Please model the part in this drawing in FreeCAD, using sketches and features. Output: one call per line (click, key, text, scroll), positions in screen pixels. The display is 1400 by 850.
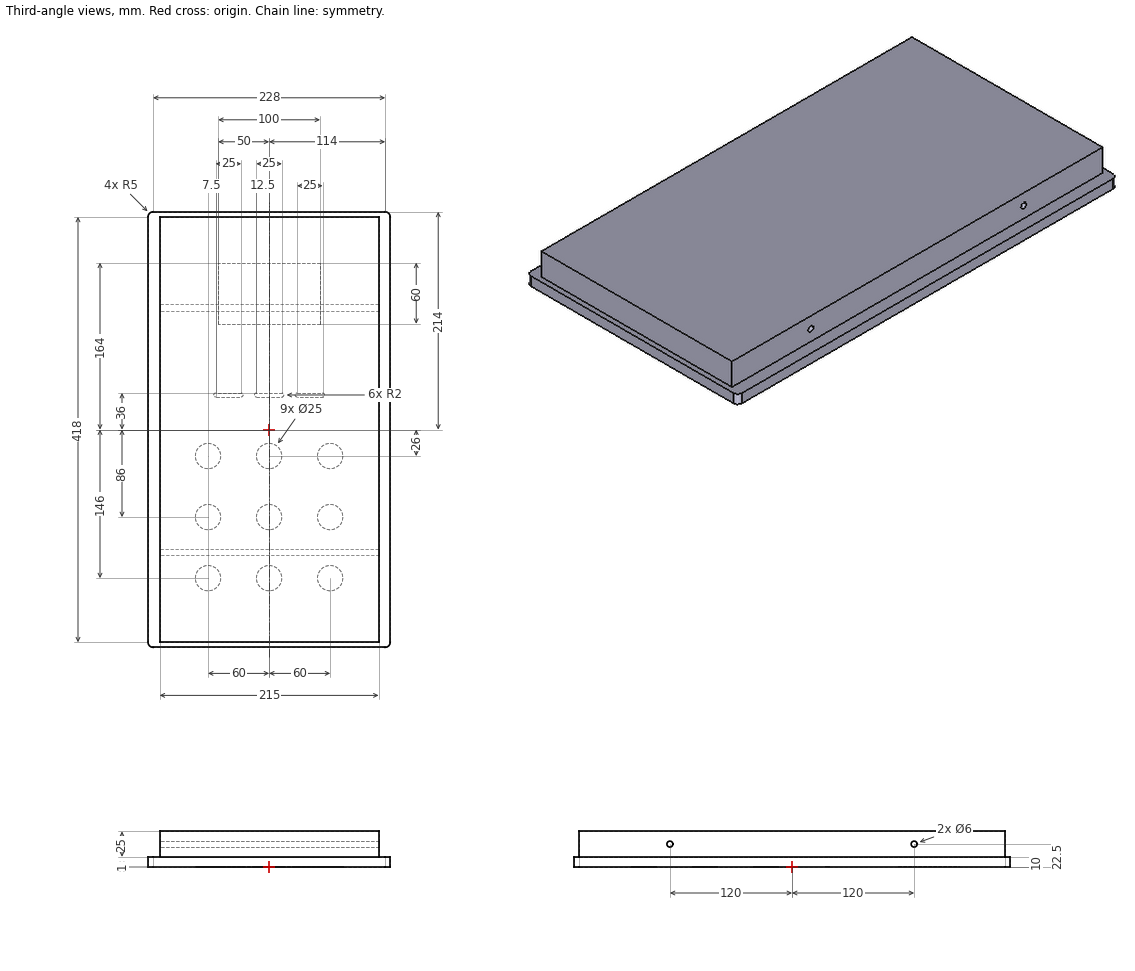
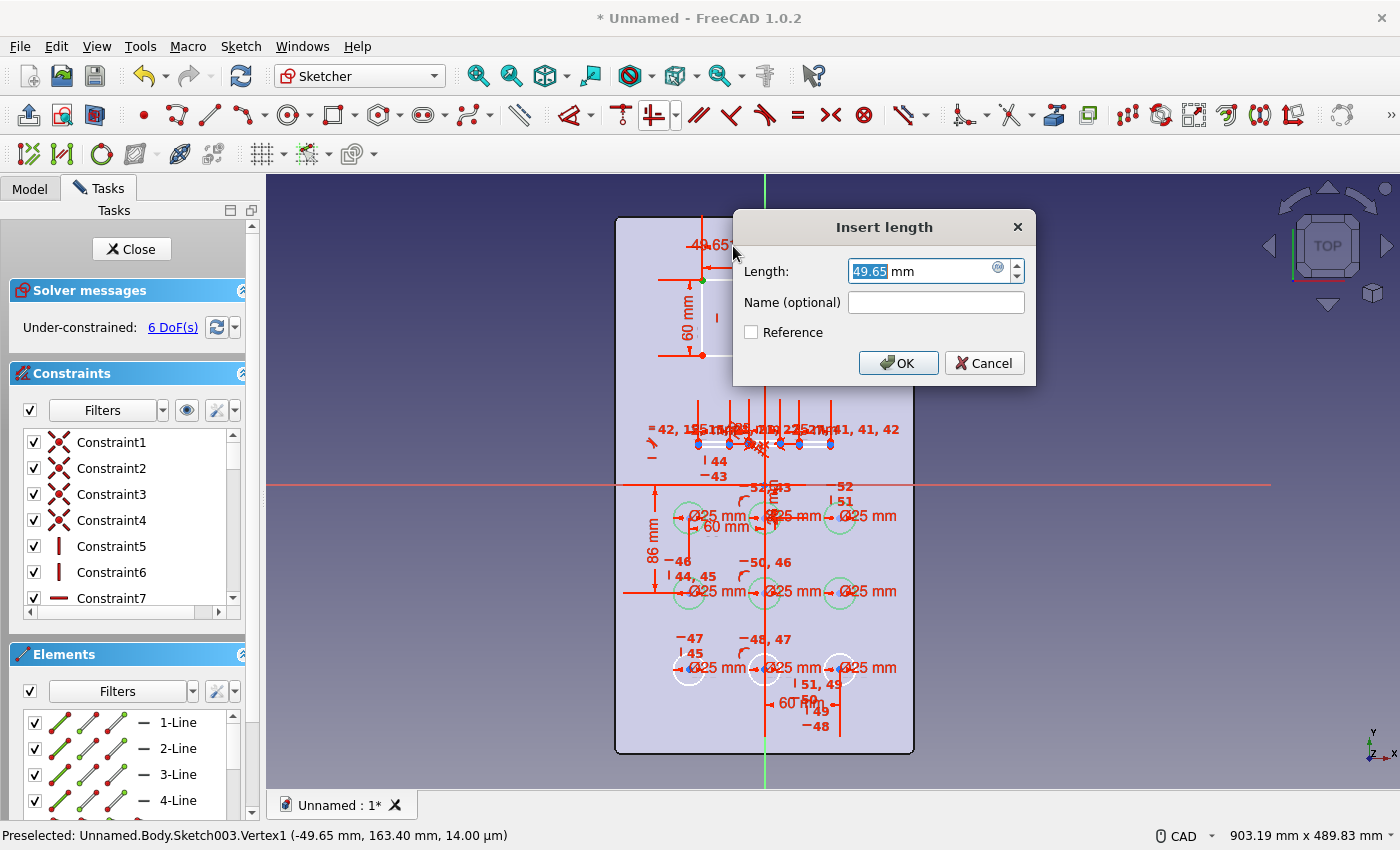
text(50)
key(Return)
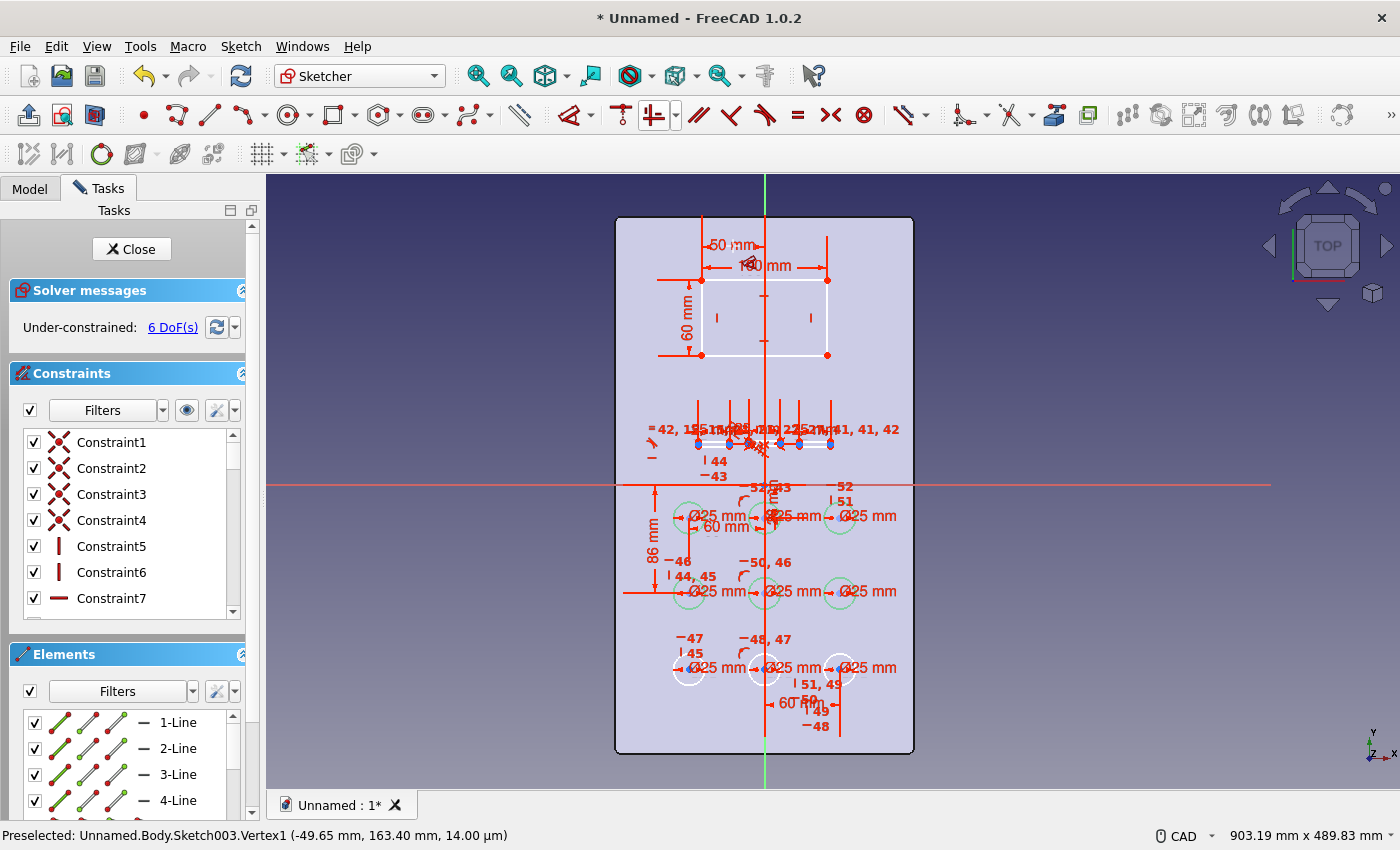
scroll(749, 441, up, 8)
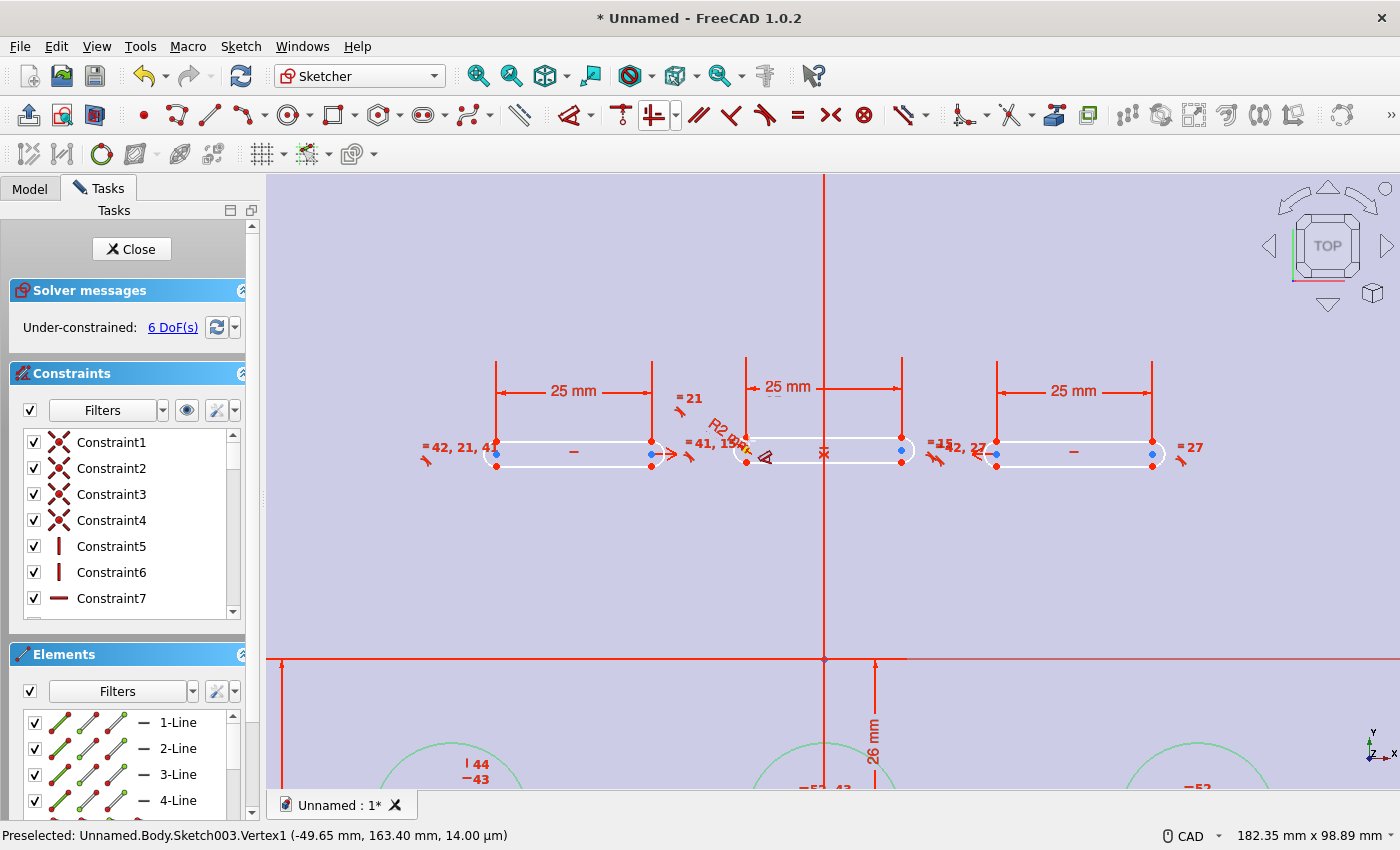
click(746, 438)
click(712, 549)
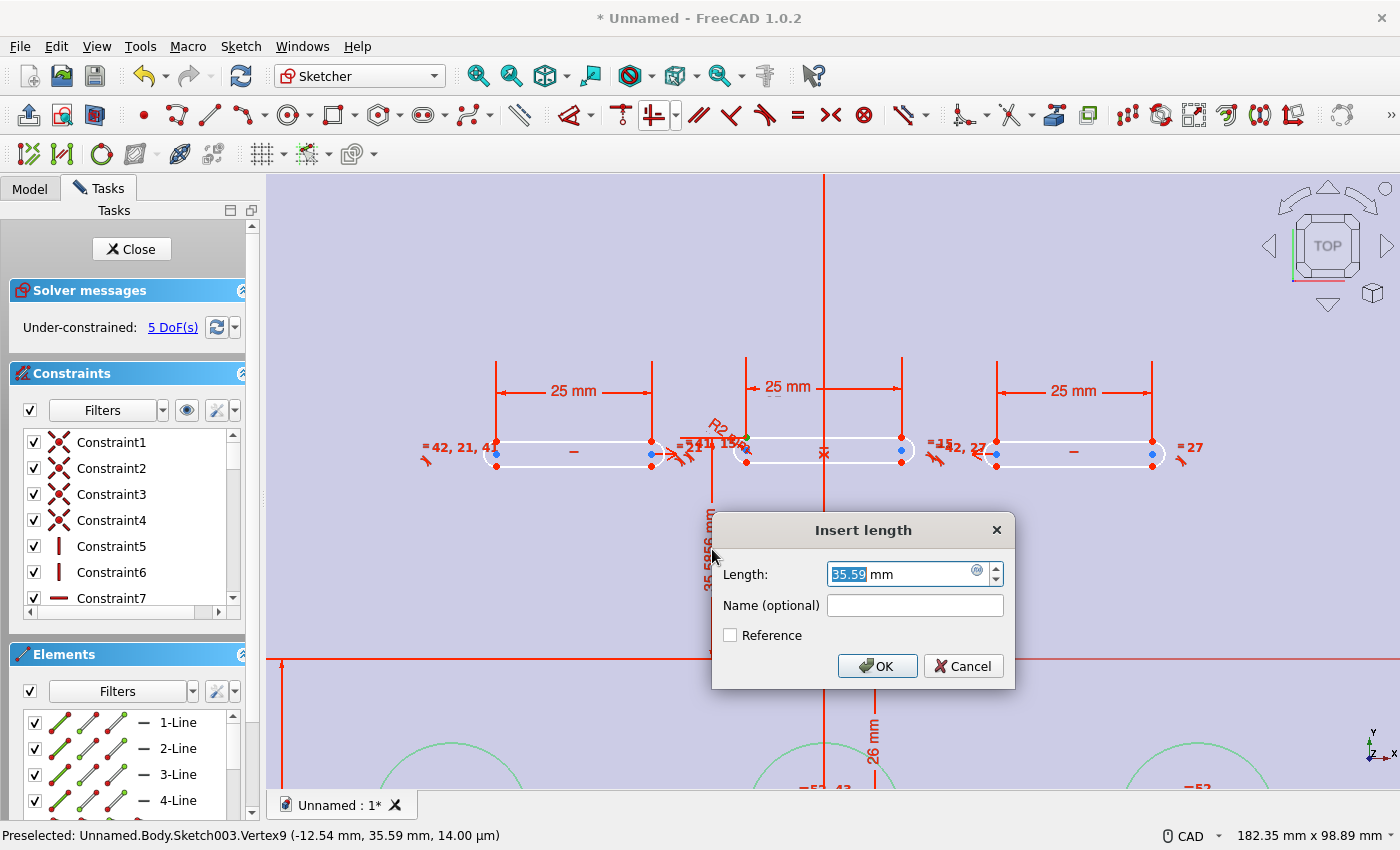
text(36)
key(Return)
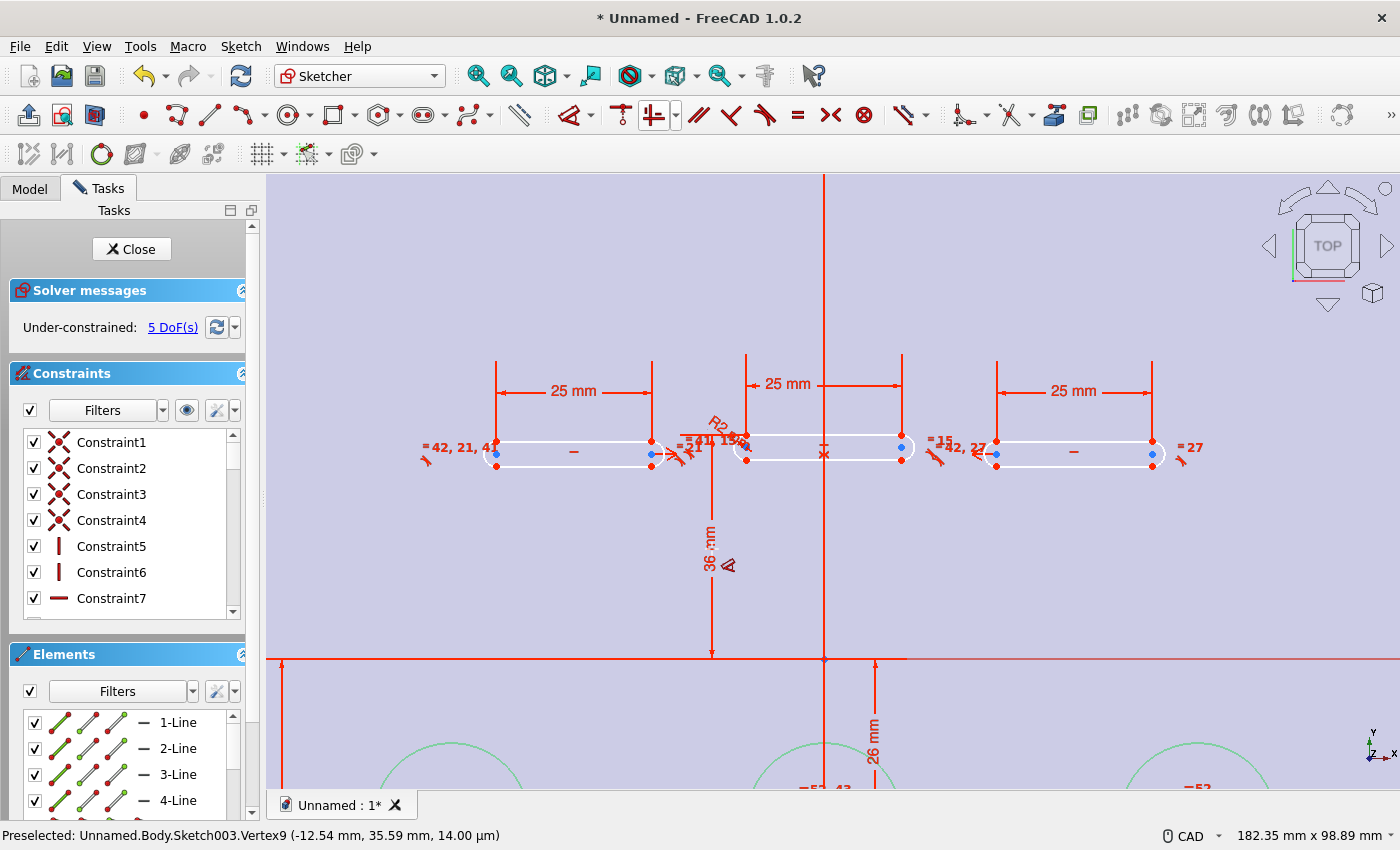
click(496, 442)
click(462, 551)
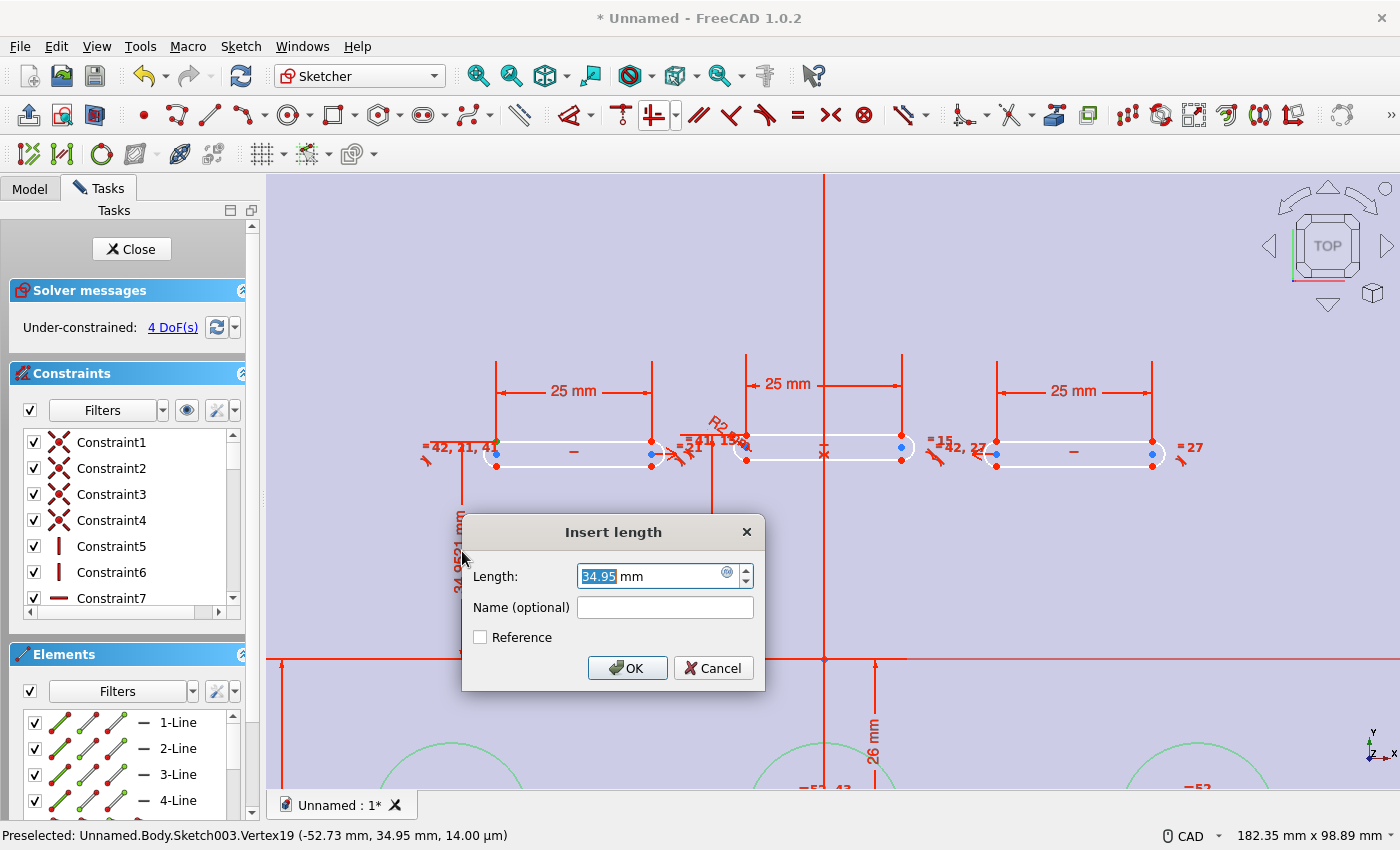
text(36)
key(Return)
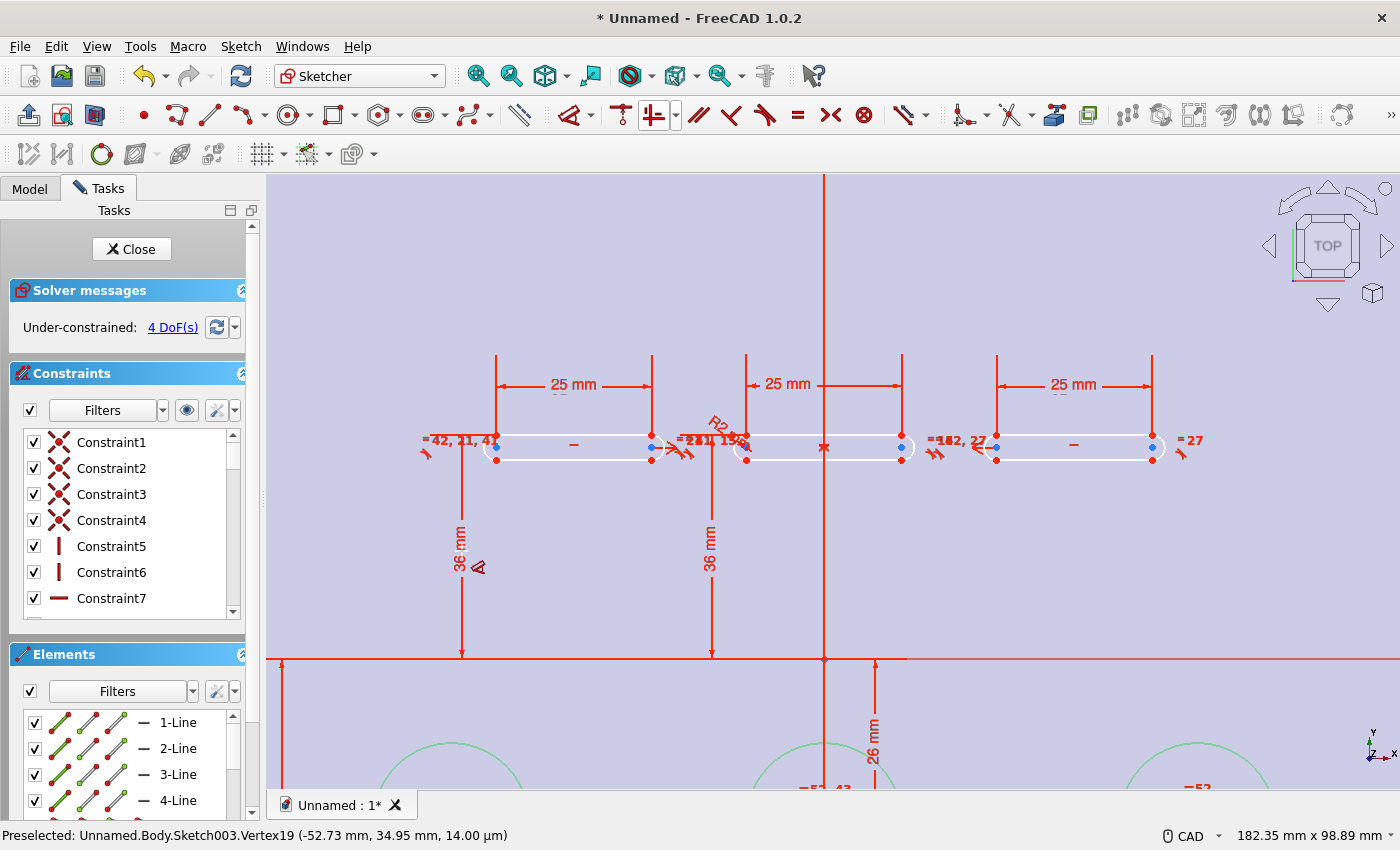
scroll(749, 441, down, 8)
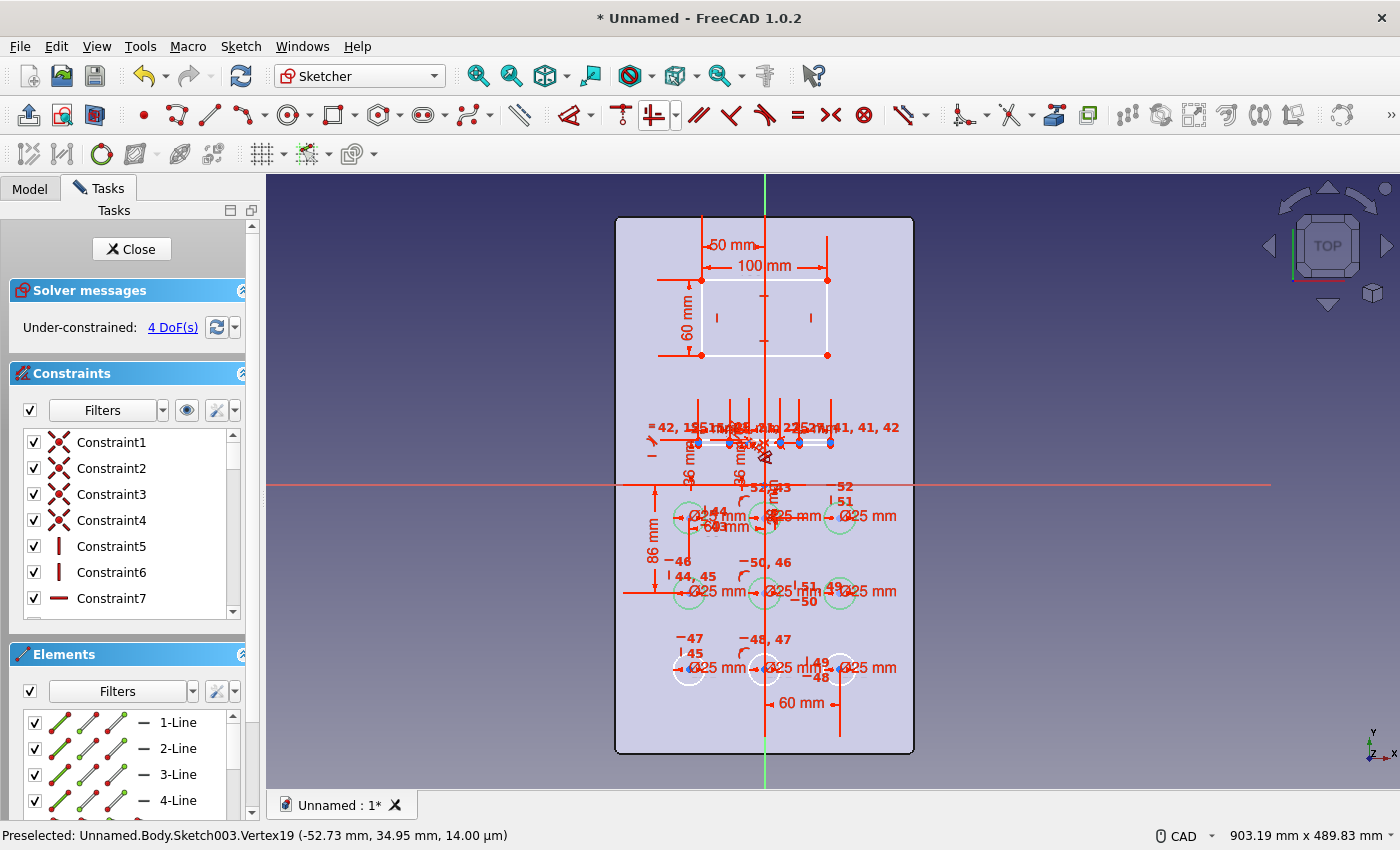
click(689, 670)
click(655, 578)